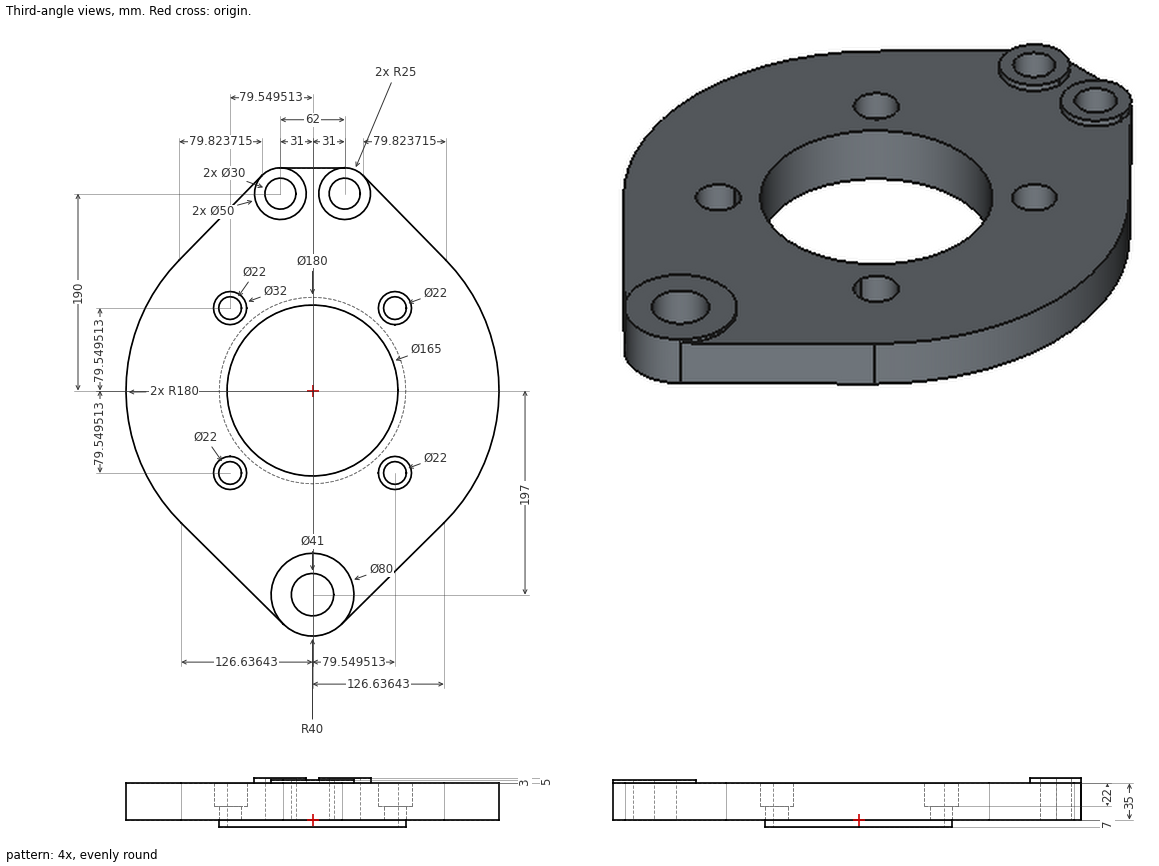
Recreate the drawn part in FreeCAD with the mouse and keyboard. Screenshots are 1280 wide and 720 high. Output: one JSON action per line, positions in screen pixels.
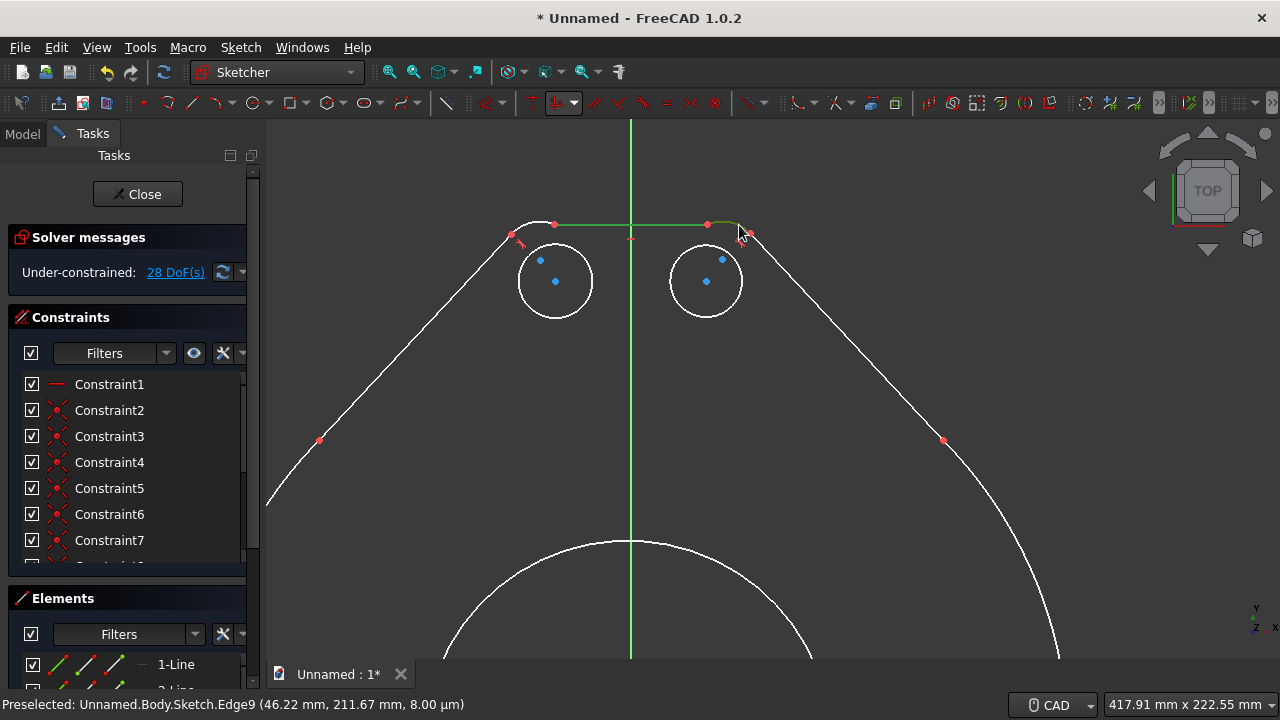
{"action": "key", "text": "t"}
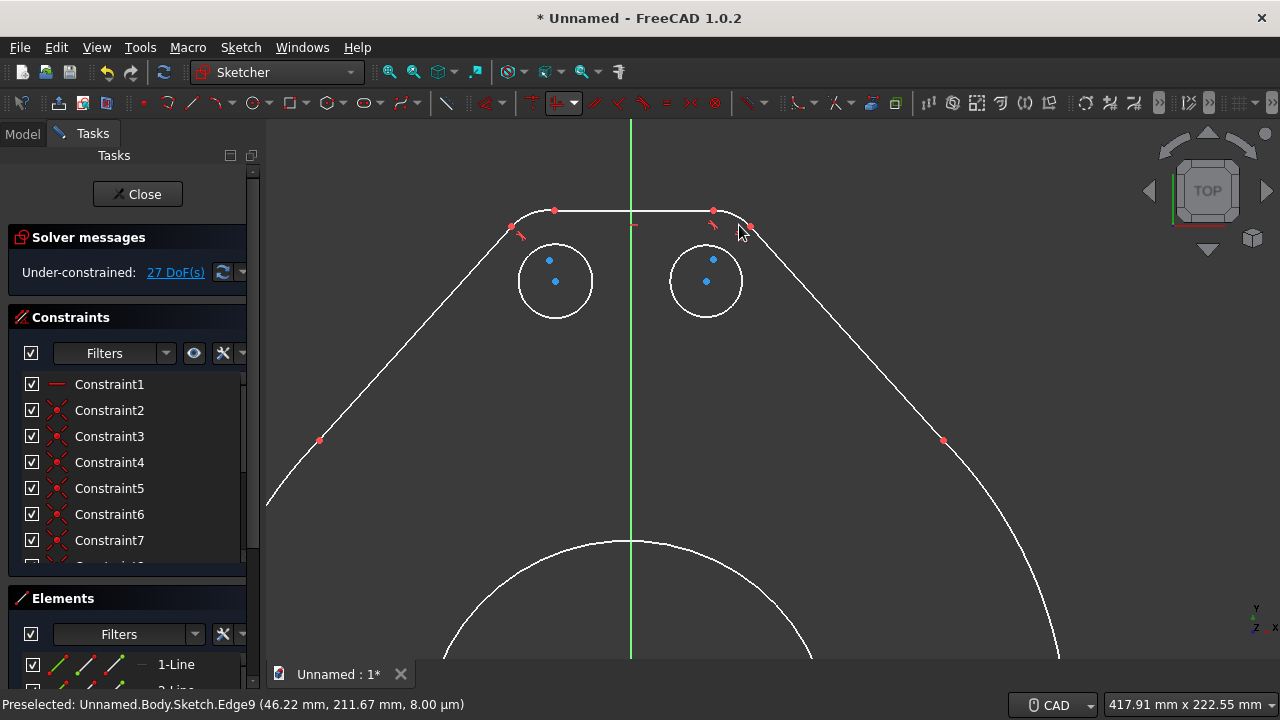
{"action": "left_click", "coordinate": [666, 211]}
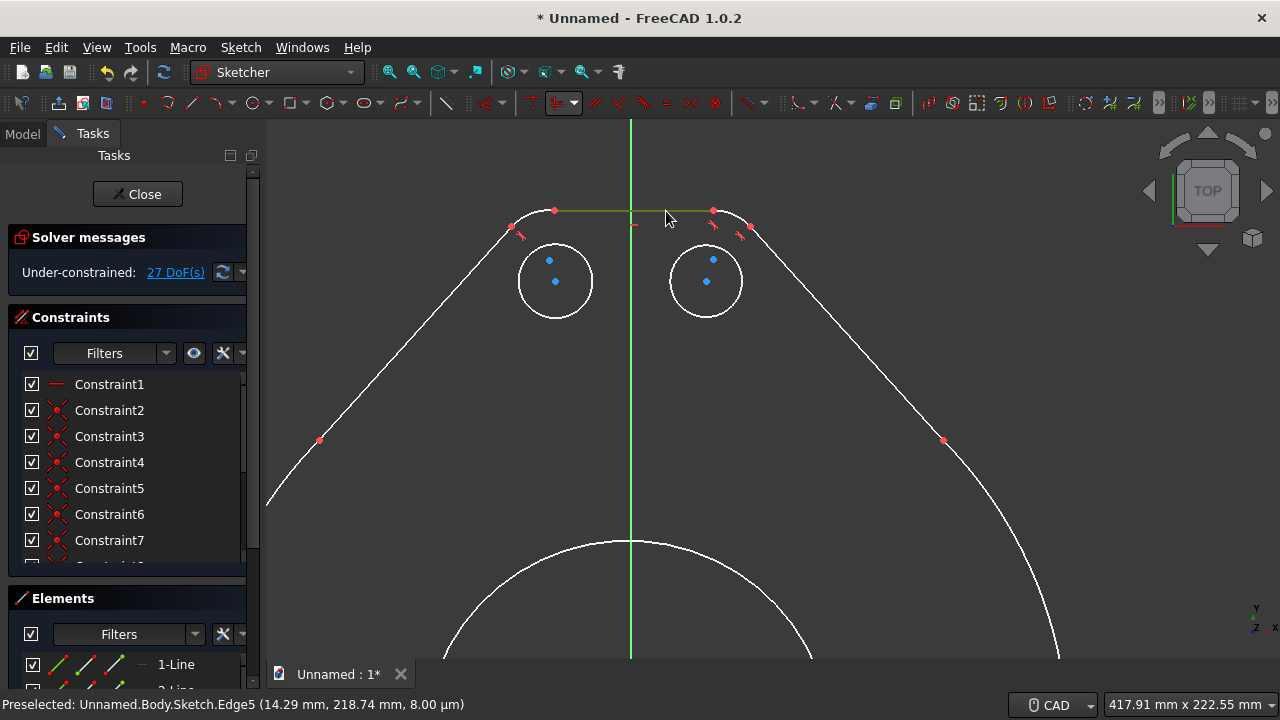
{"action": "left_click", "coordinate": [540, 211]}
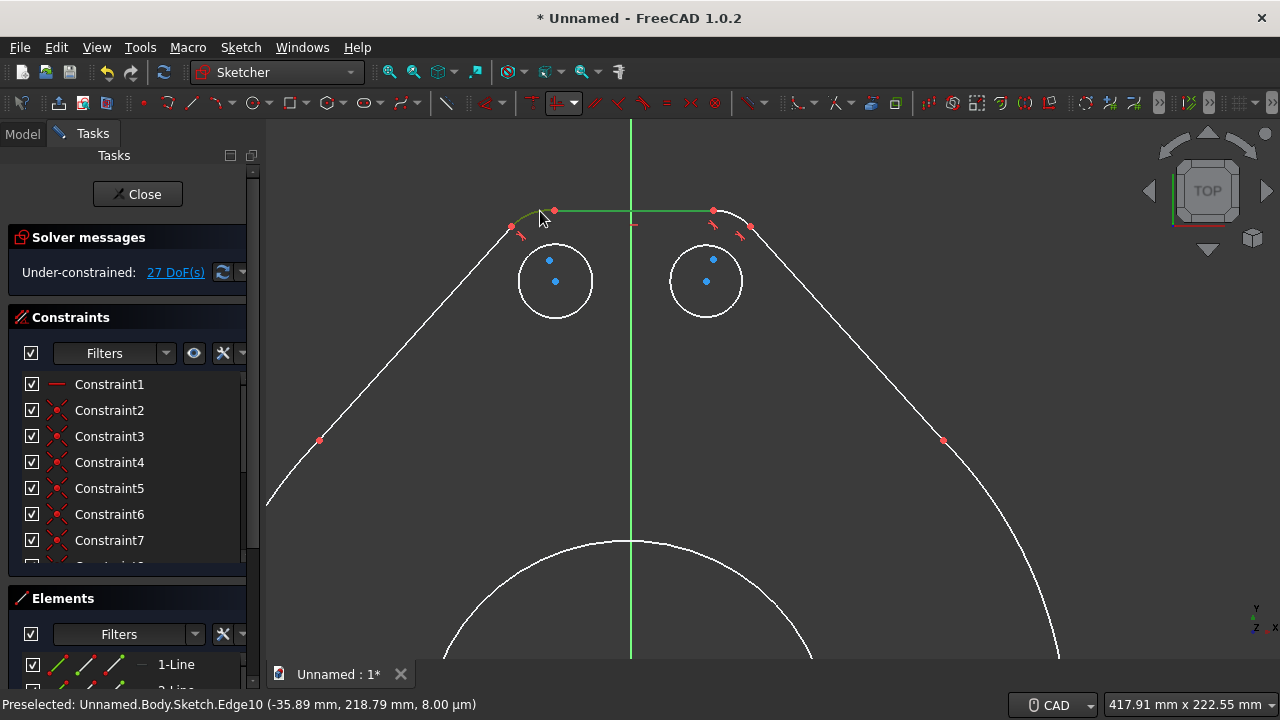
{"action": "key", "text": "t"}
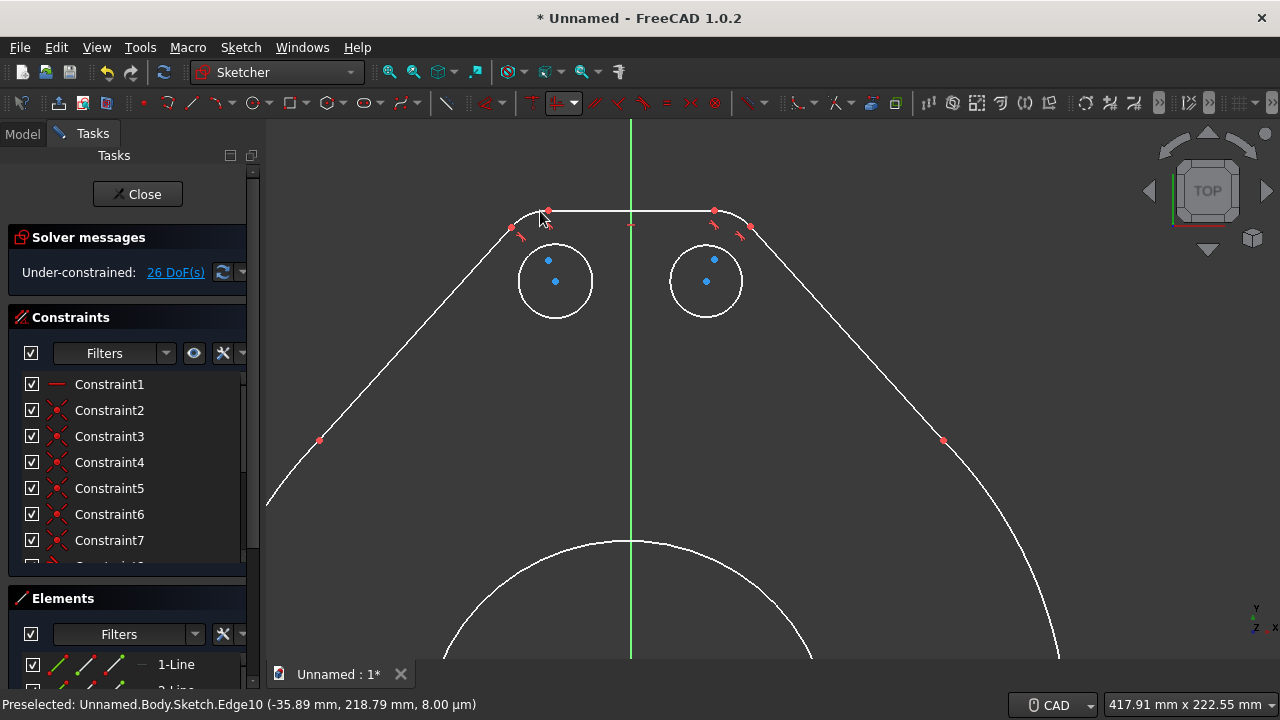
{"action": "left_click", "coordinate": [771, 600]}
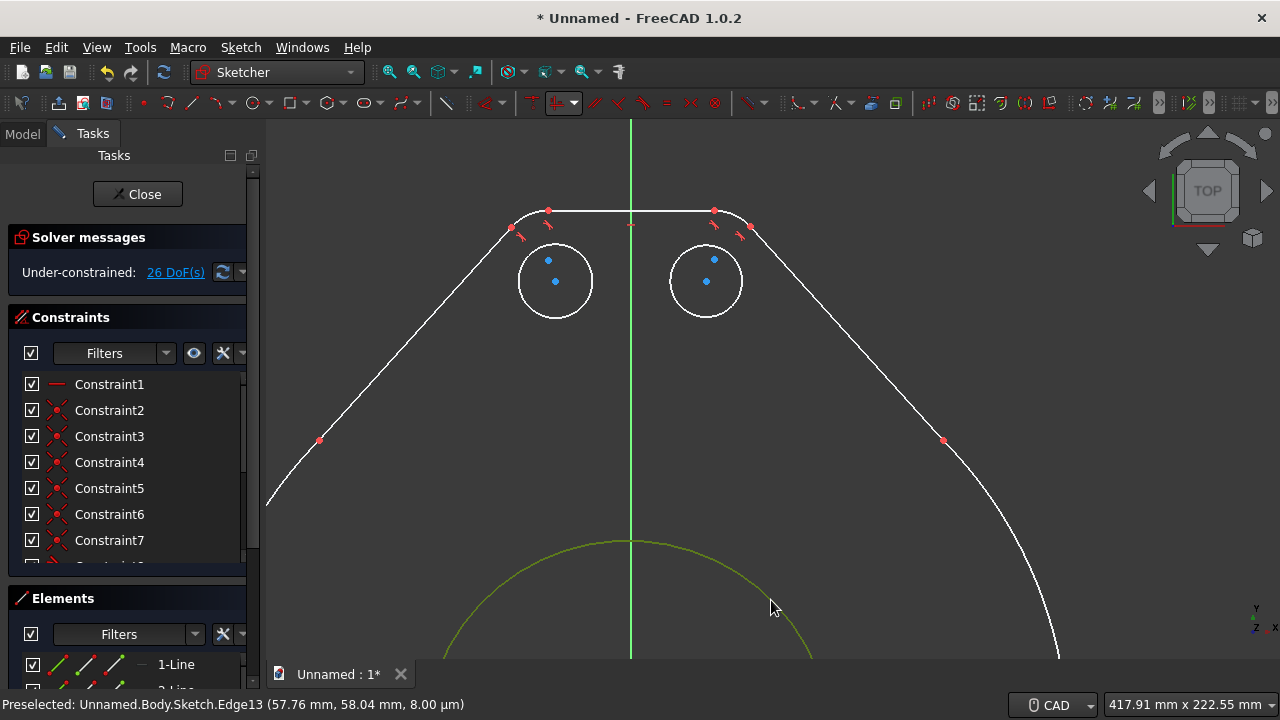
{"action": "left_click", "coordinate": [1048, 614]}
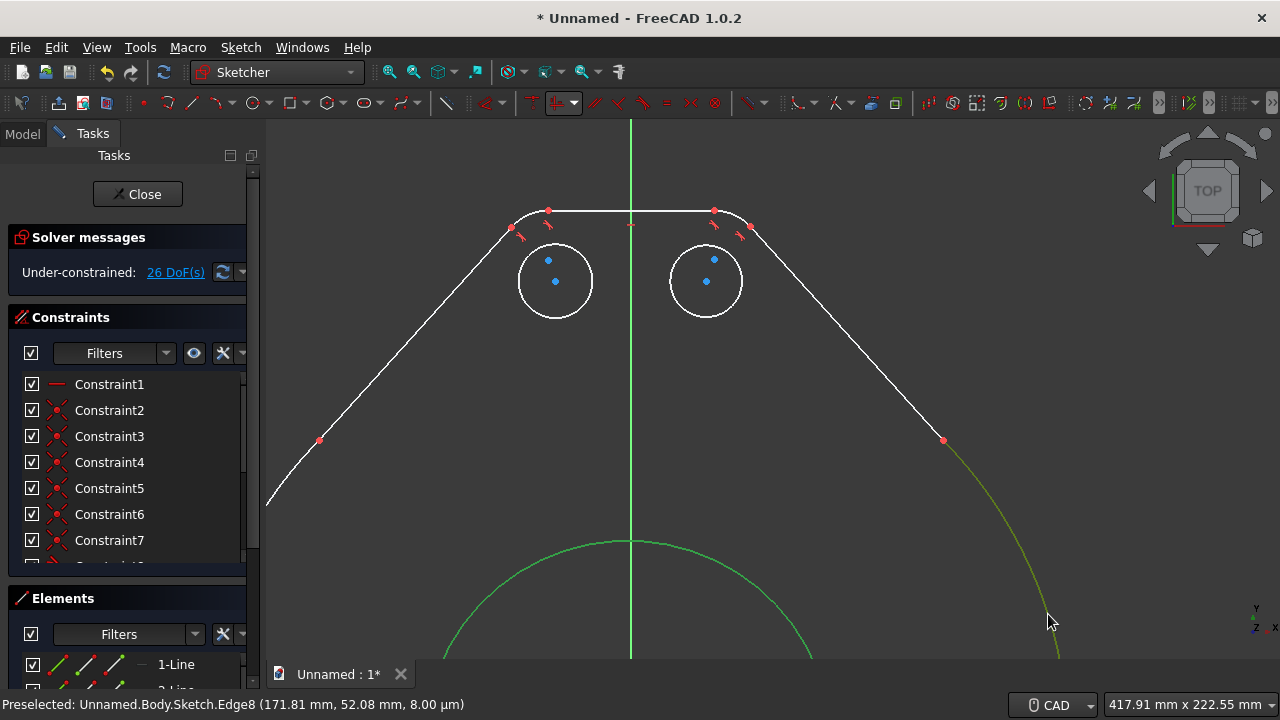
{"action": "key", "text": "c"}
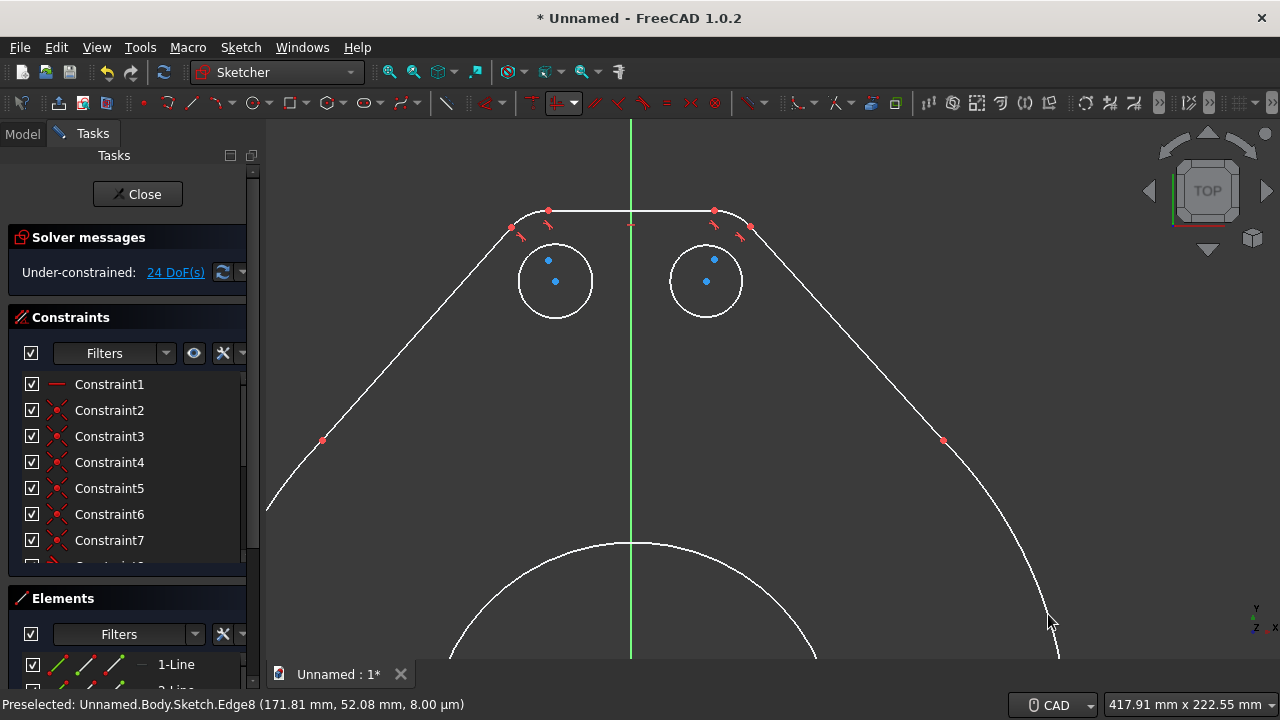
{"action": "left_click", "coordinate": [731, 256]}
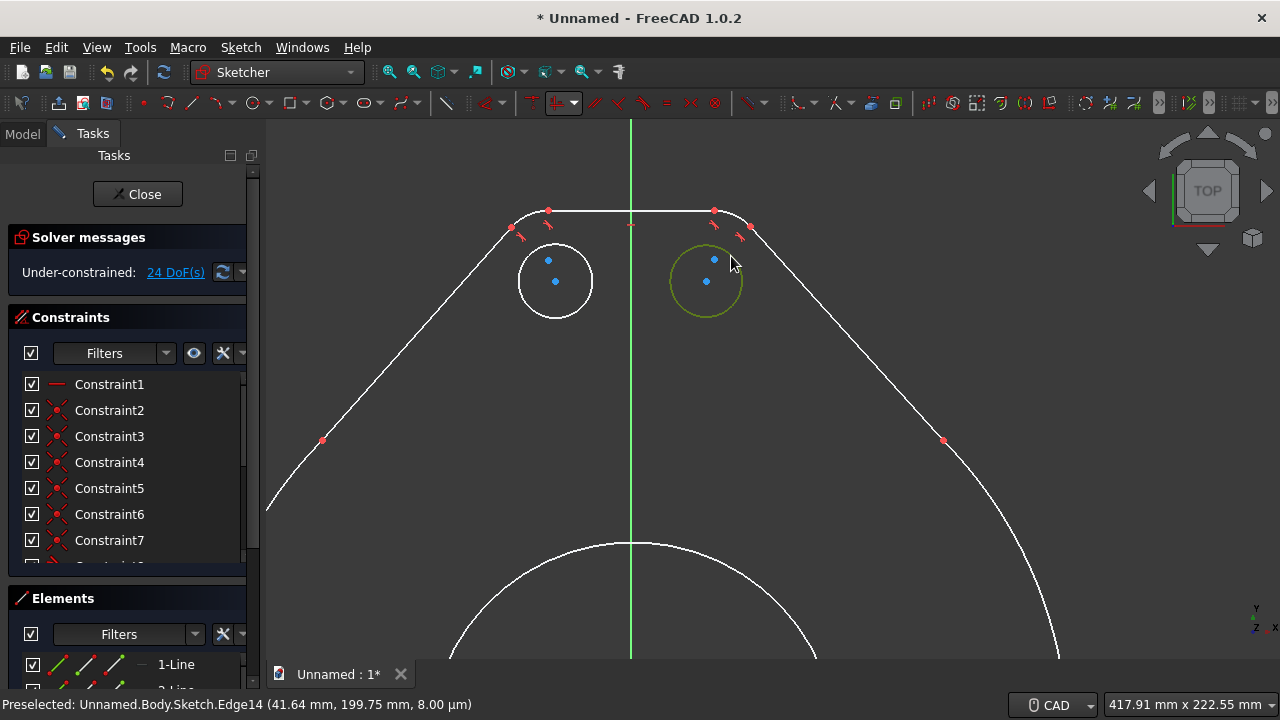
{"action": "left_click", "coordinate": [741, 219]}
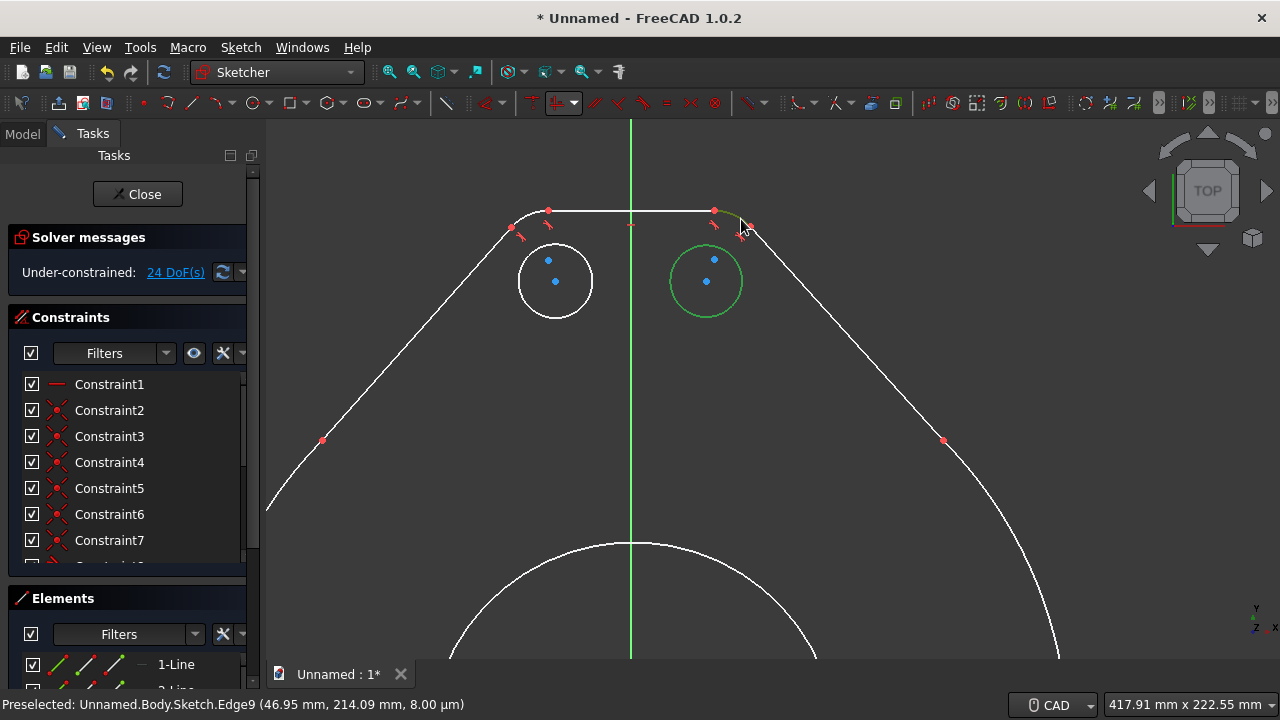
{"action": "key", "text": "c"}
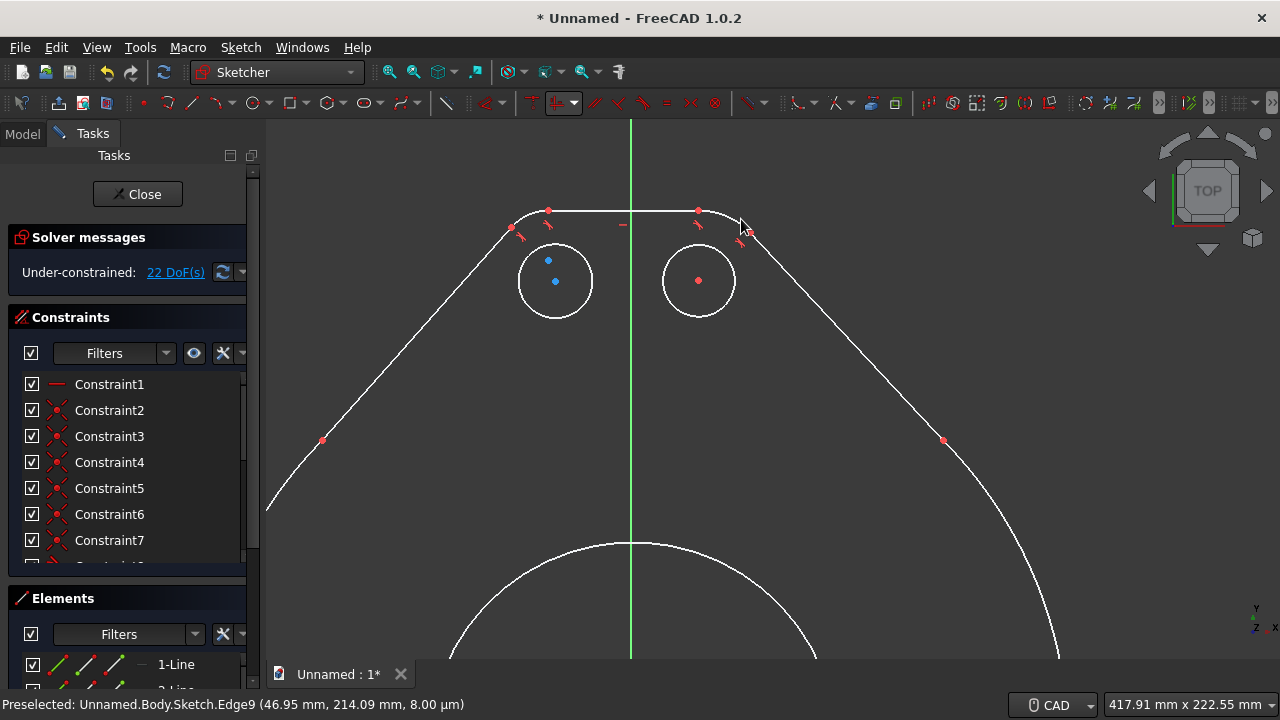
{"action": "left_click", "coordinate": [582, 255]}